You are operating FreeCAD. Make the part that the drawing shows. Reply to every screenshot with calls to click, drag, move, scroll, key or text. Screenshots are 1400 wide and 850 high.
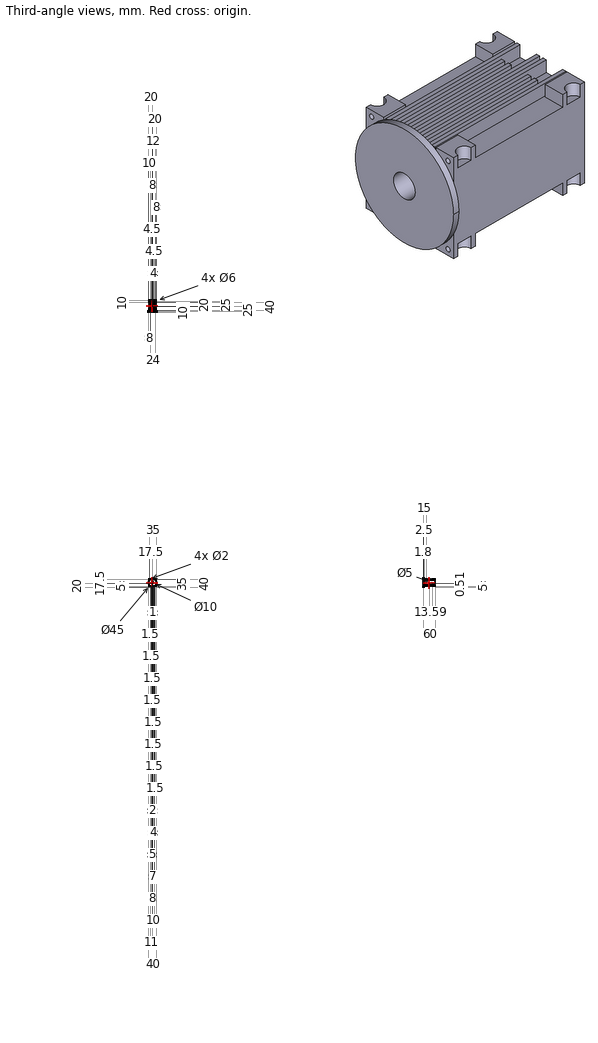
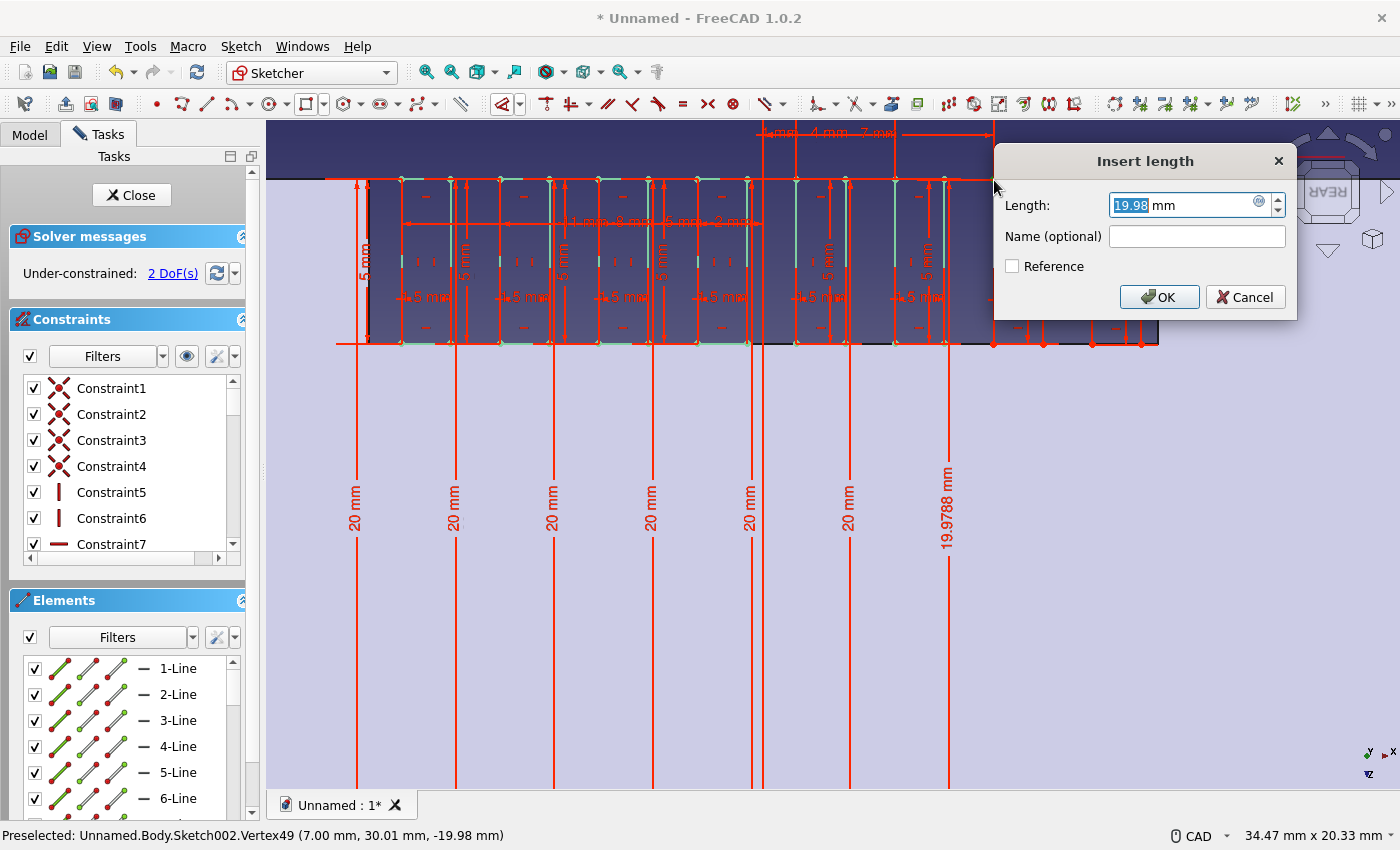
text(20)
key(Return)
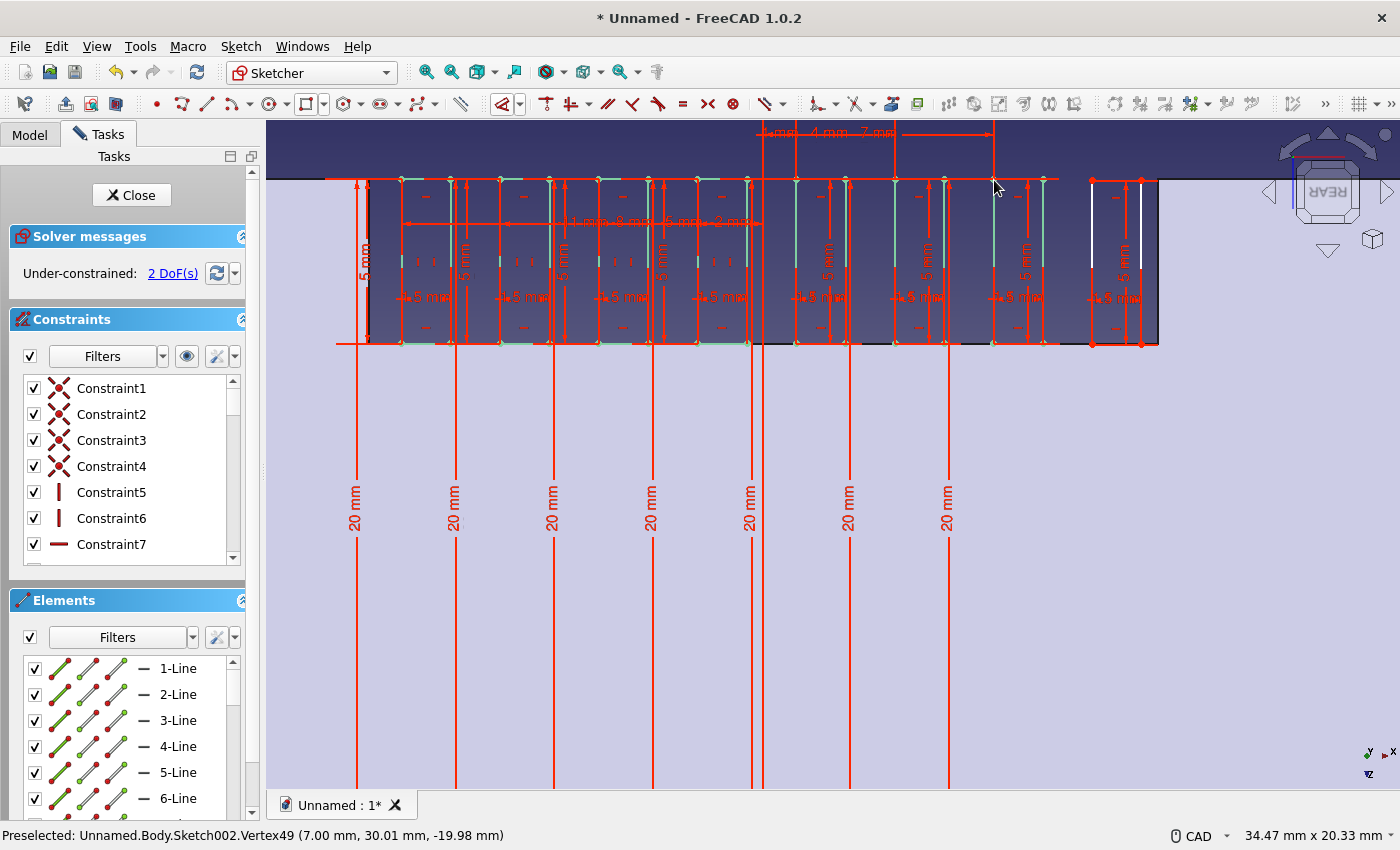
click(1092, 181)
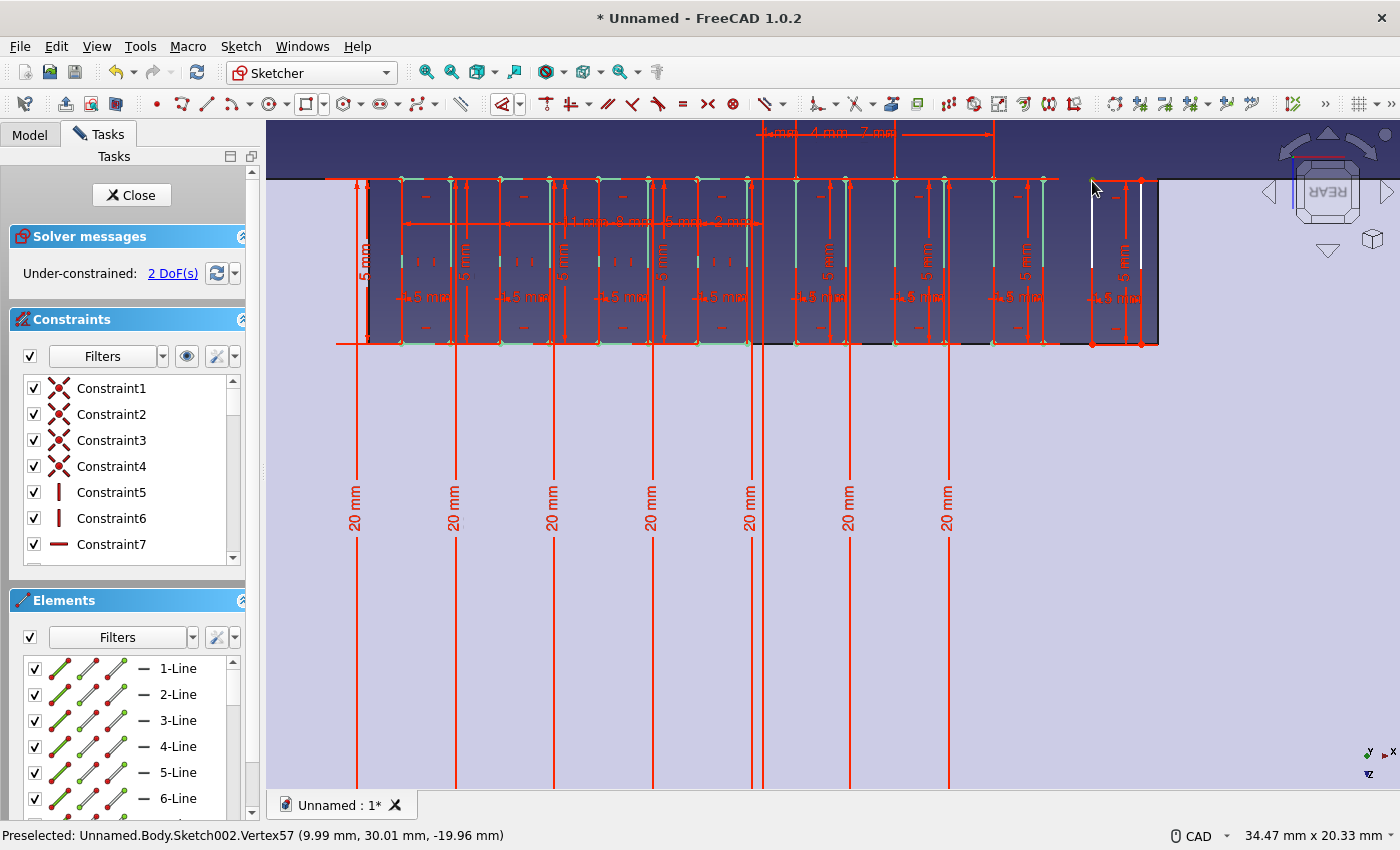
click(520, 104)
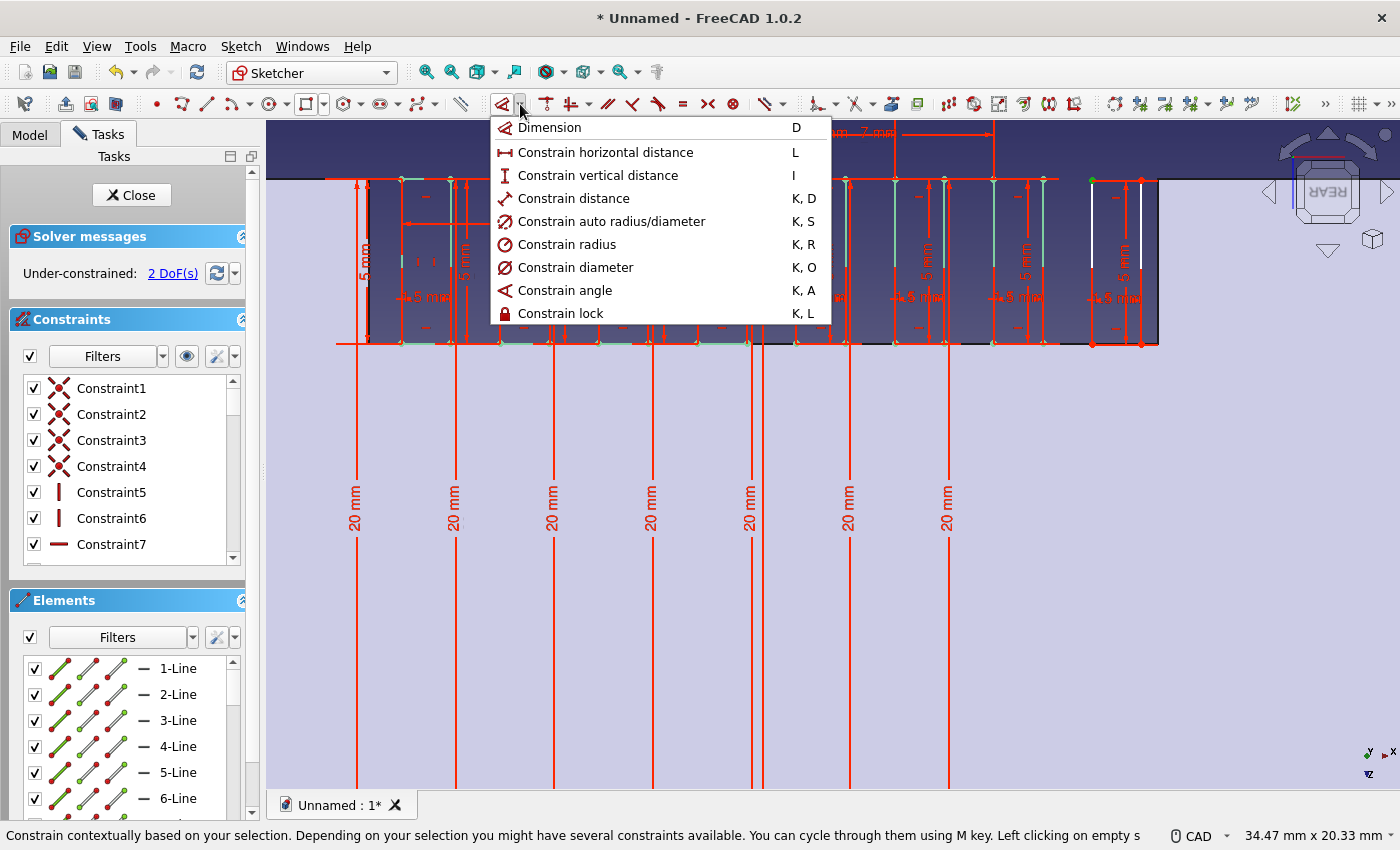
click(661, 152)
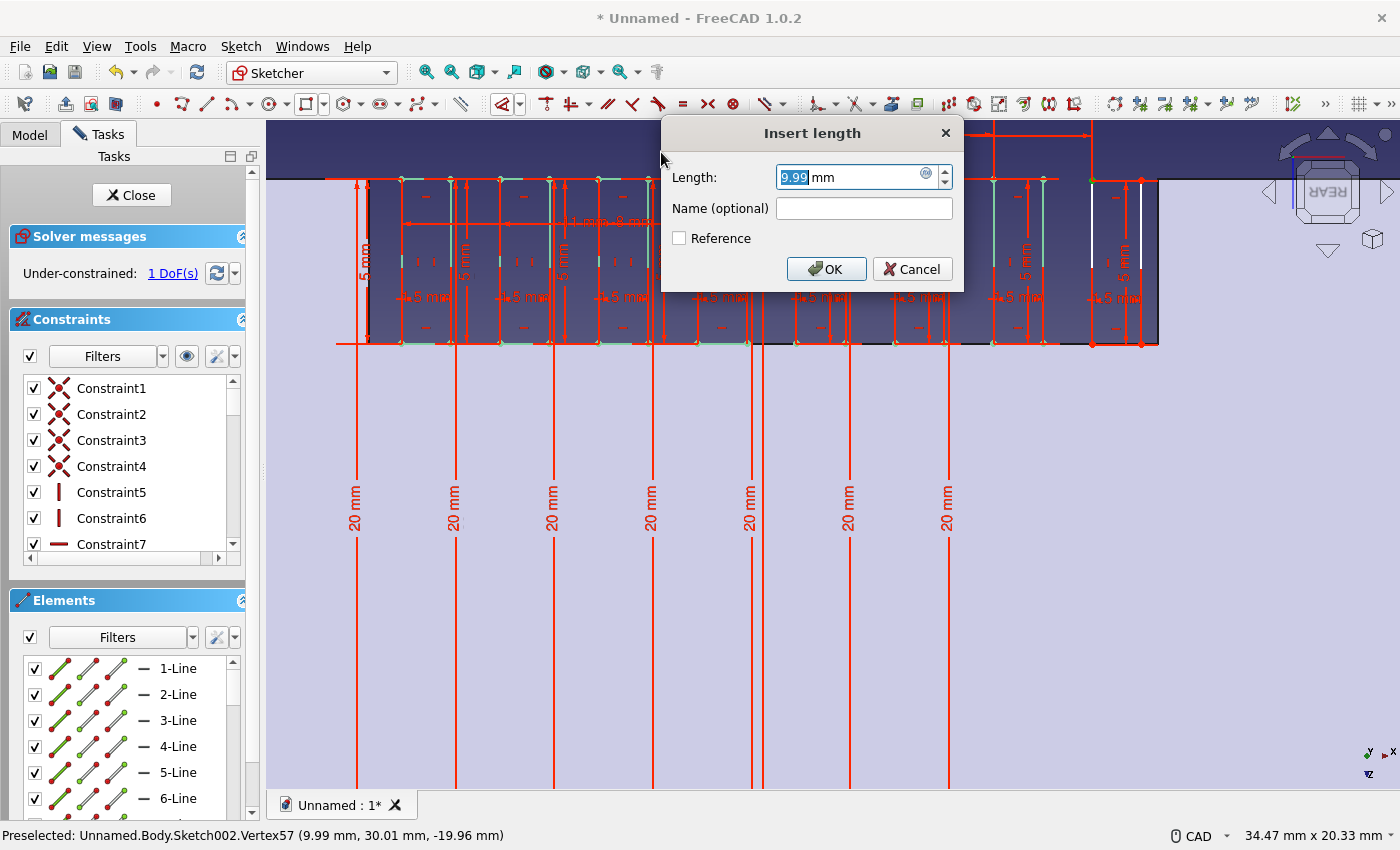
text(10)
key(Return)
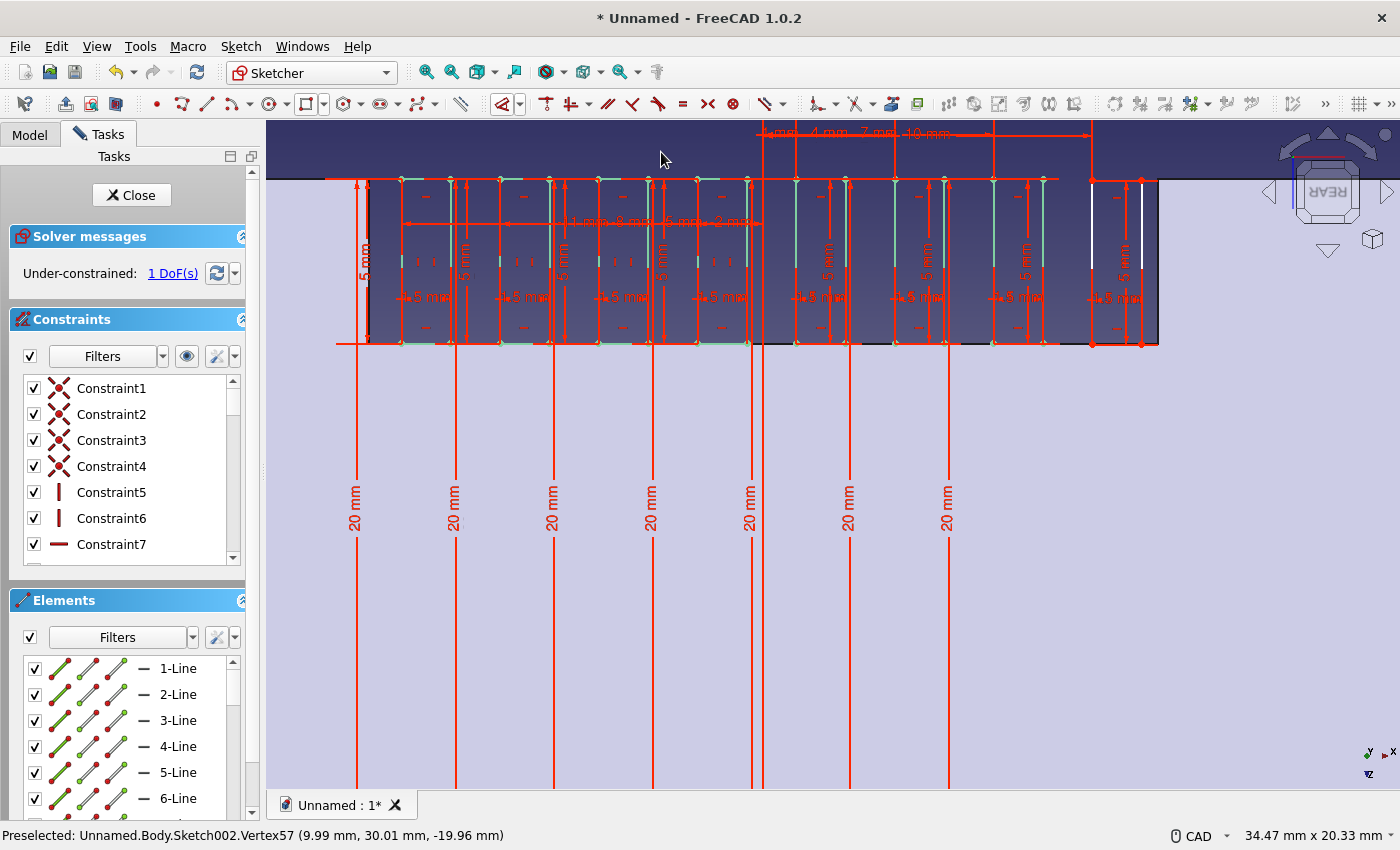
click(1092, 181)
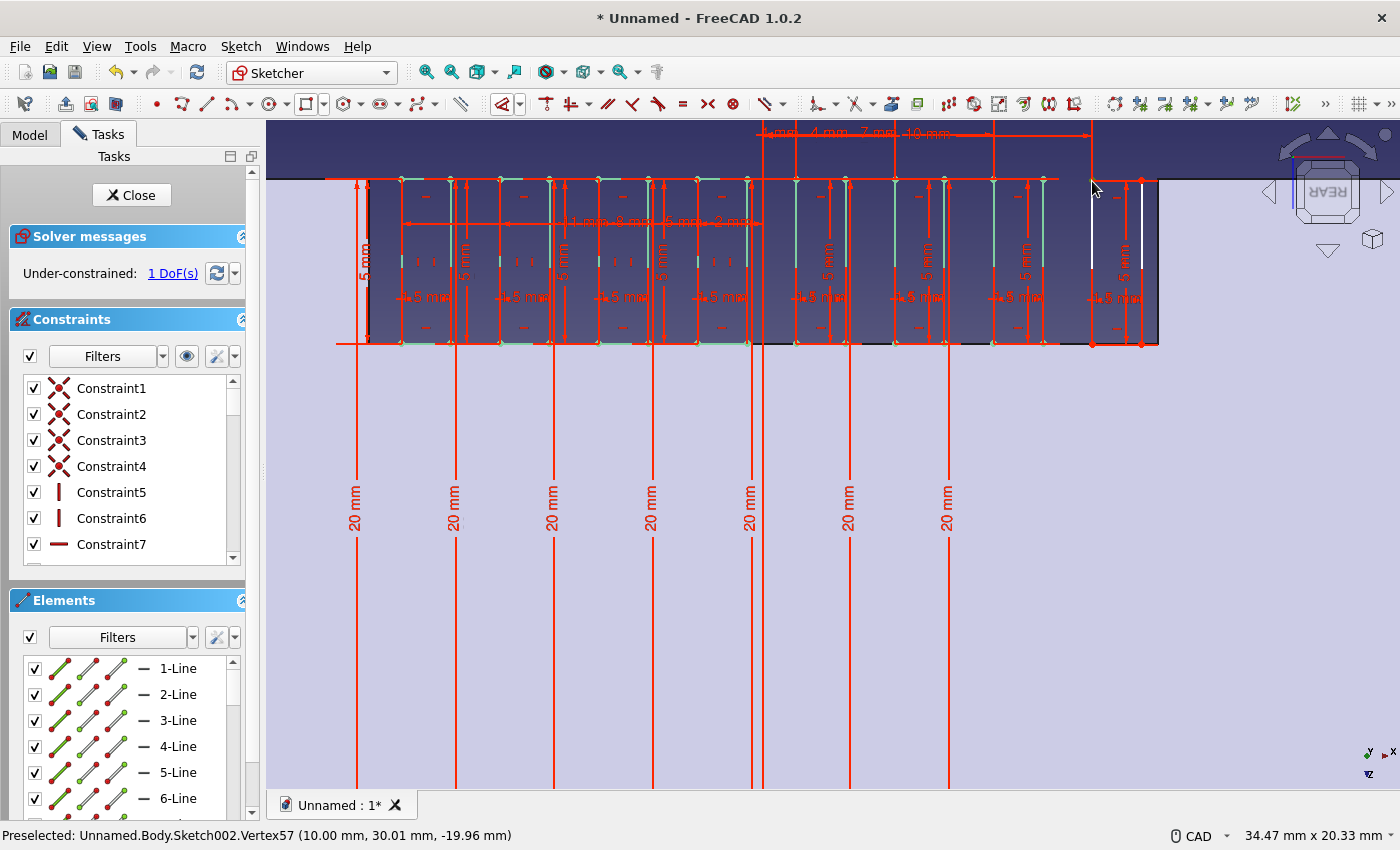
click(520, 104)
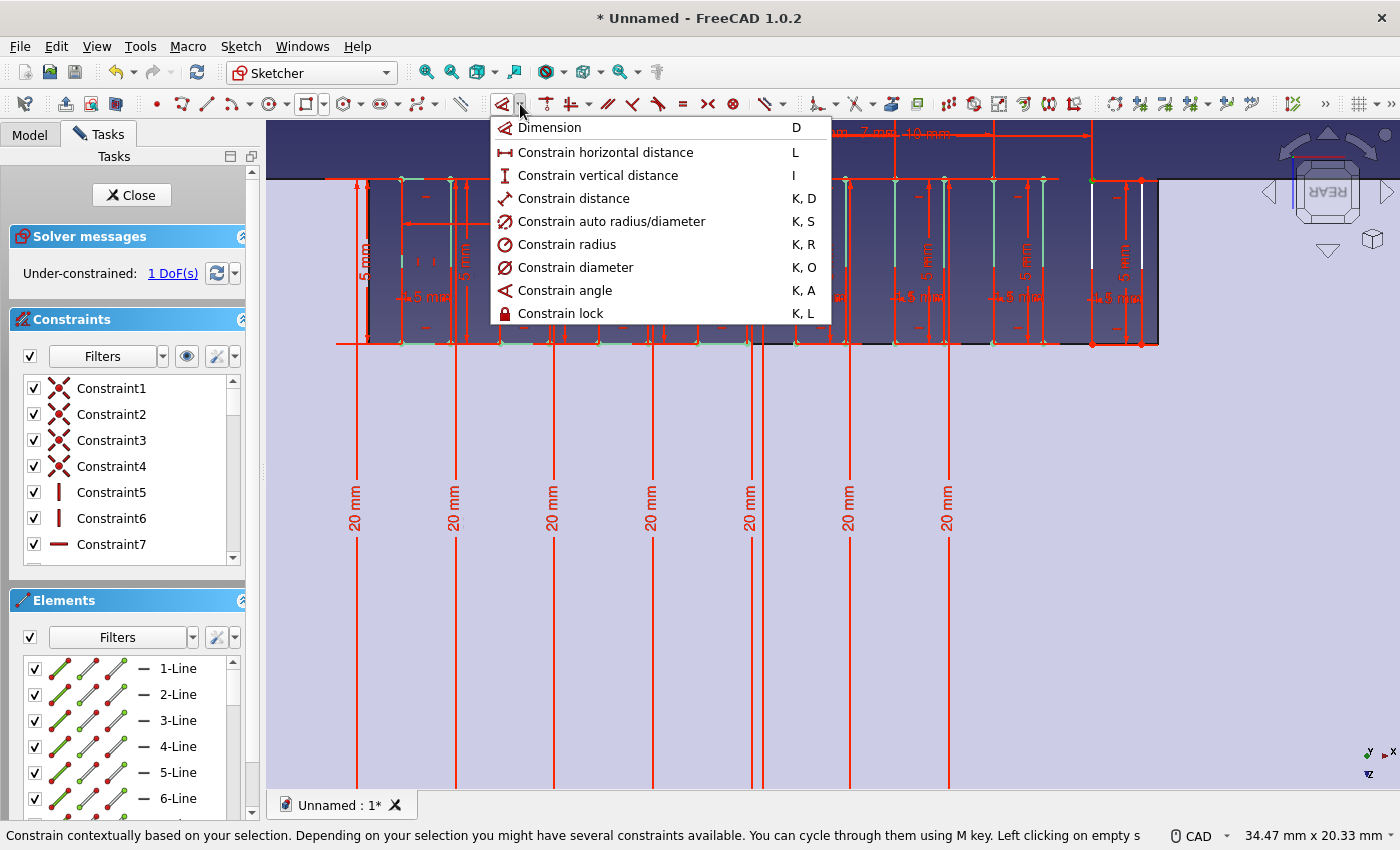
click(661, 176)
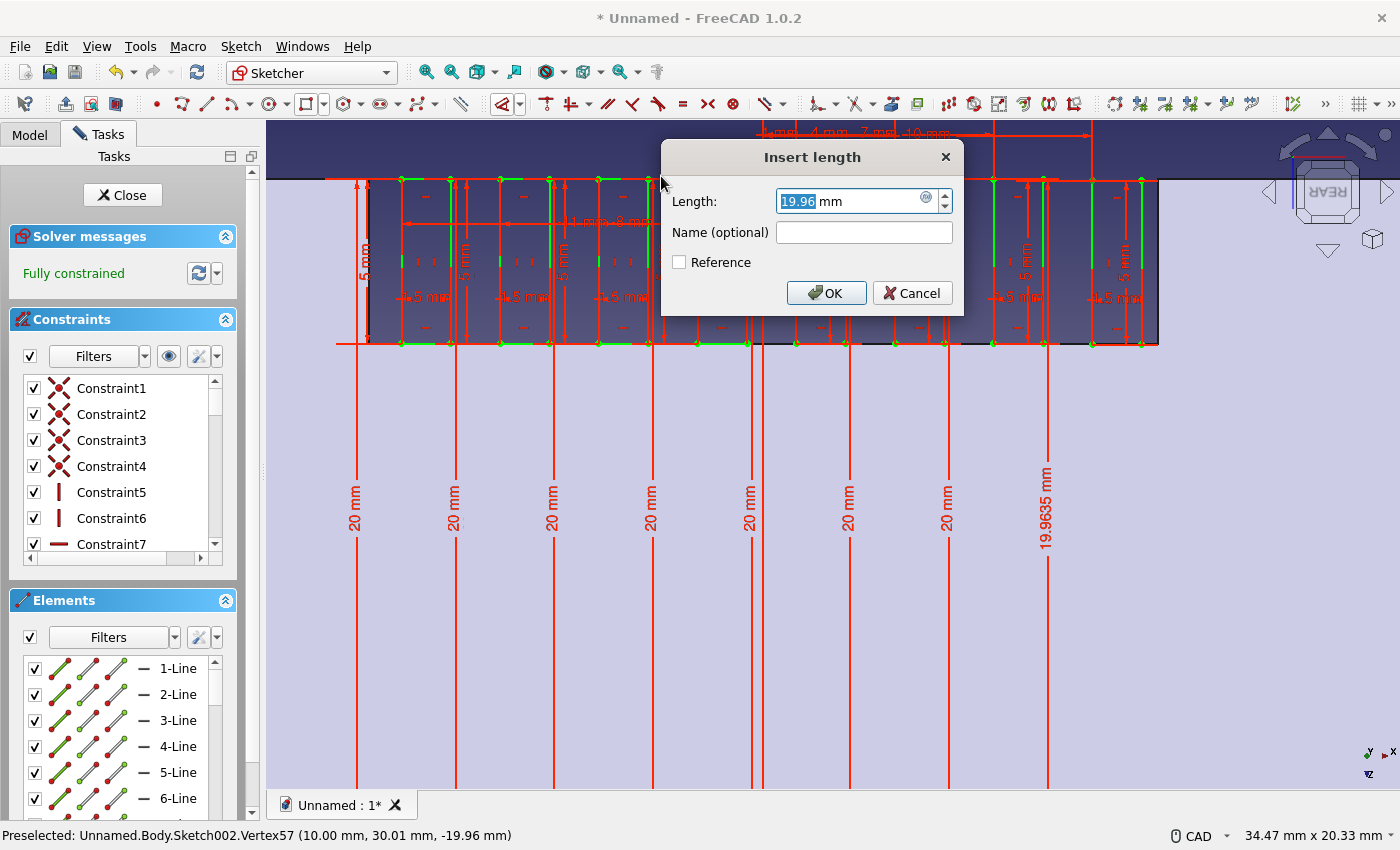
text(20)
key(Return)